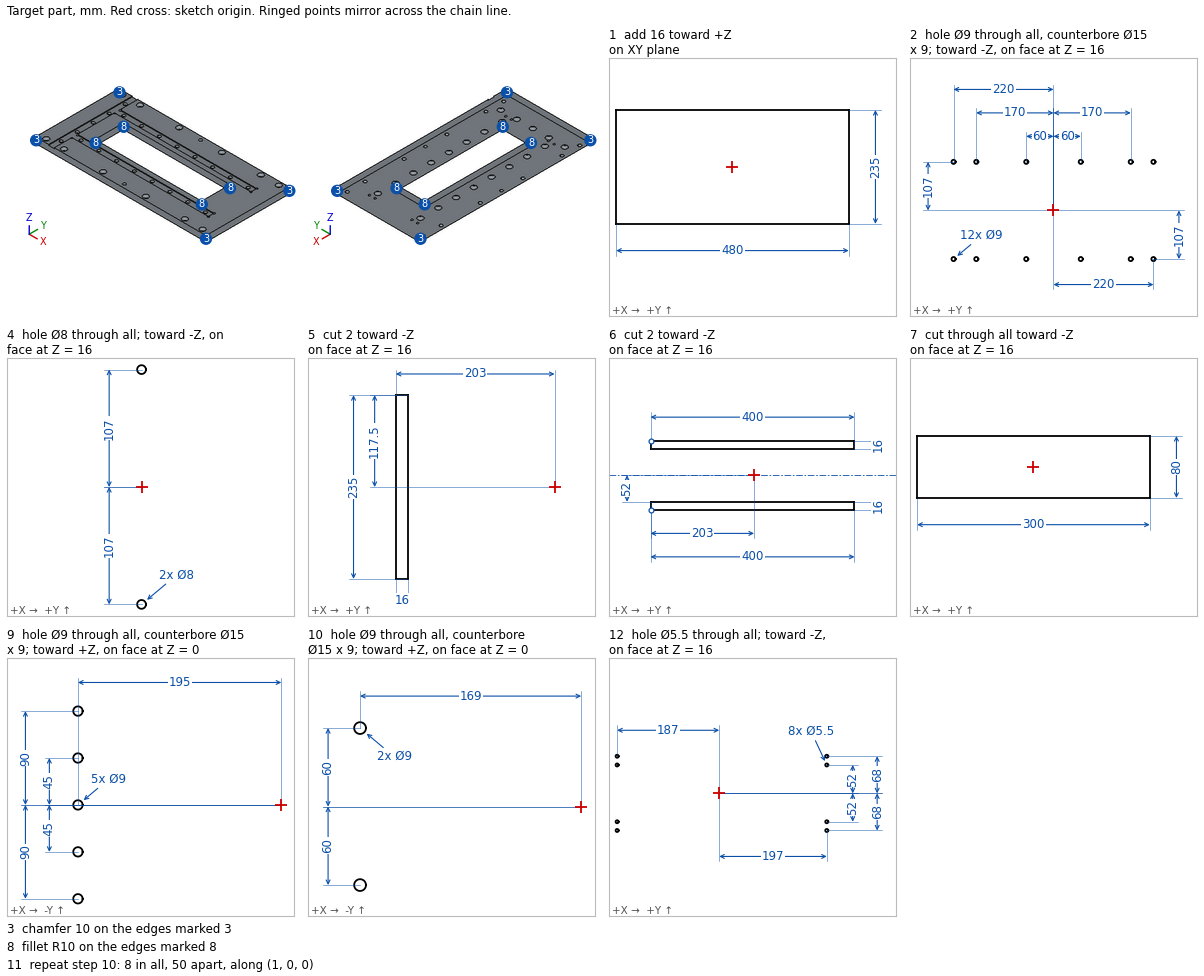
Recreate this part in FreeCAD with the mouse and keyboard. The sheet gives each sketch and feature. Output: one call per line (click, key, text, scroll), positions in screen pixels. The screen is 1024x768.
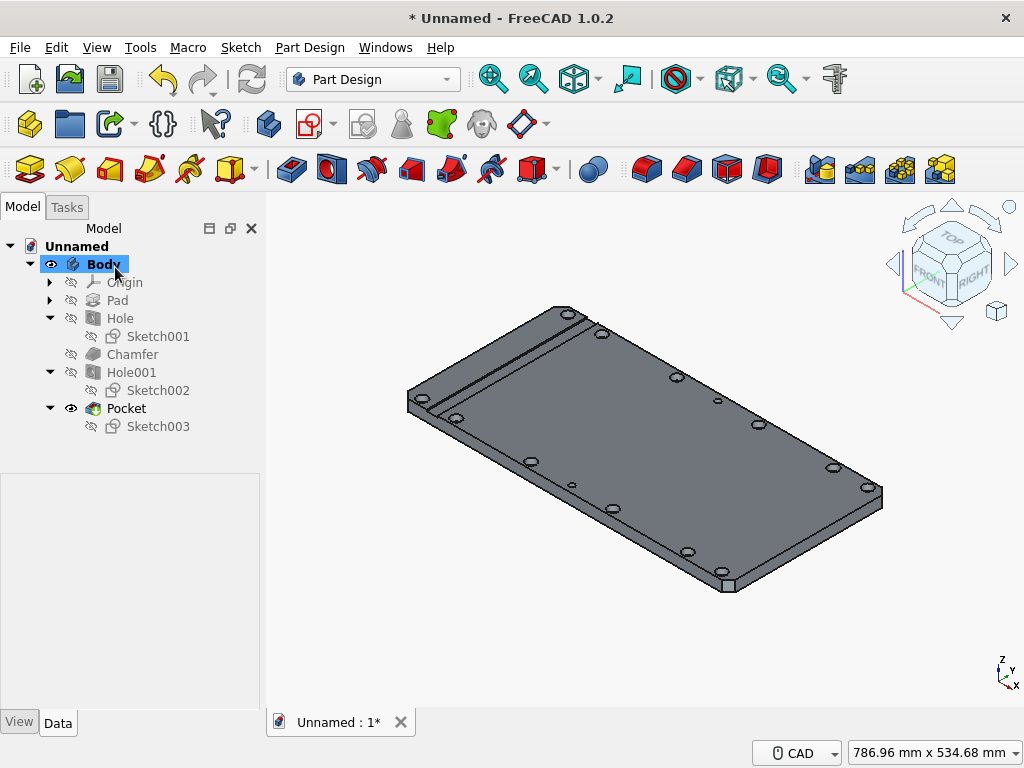
click(663, 453)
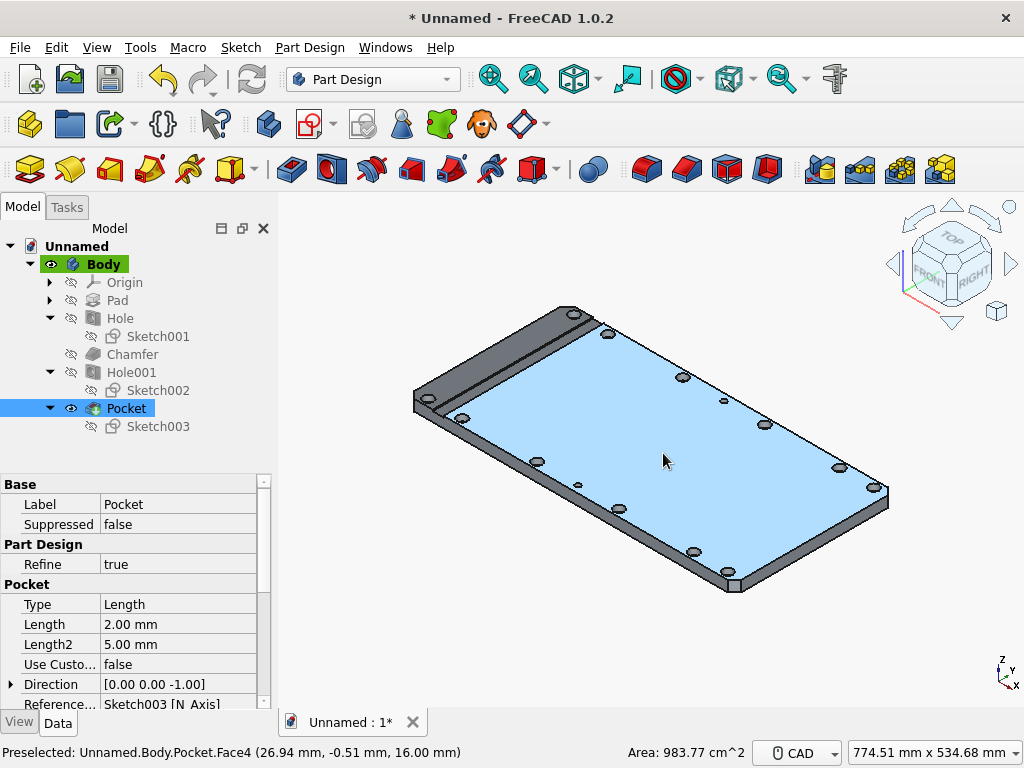
click(310, 124)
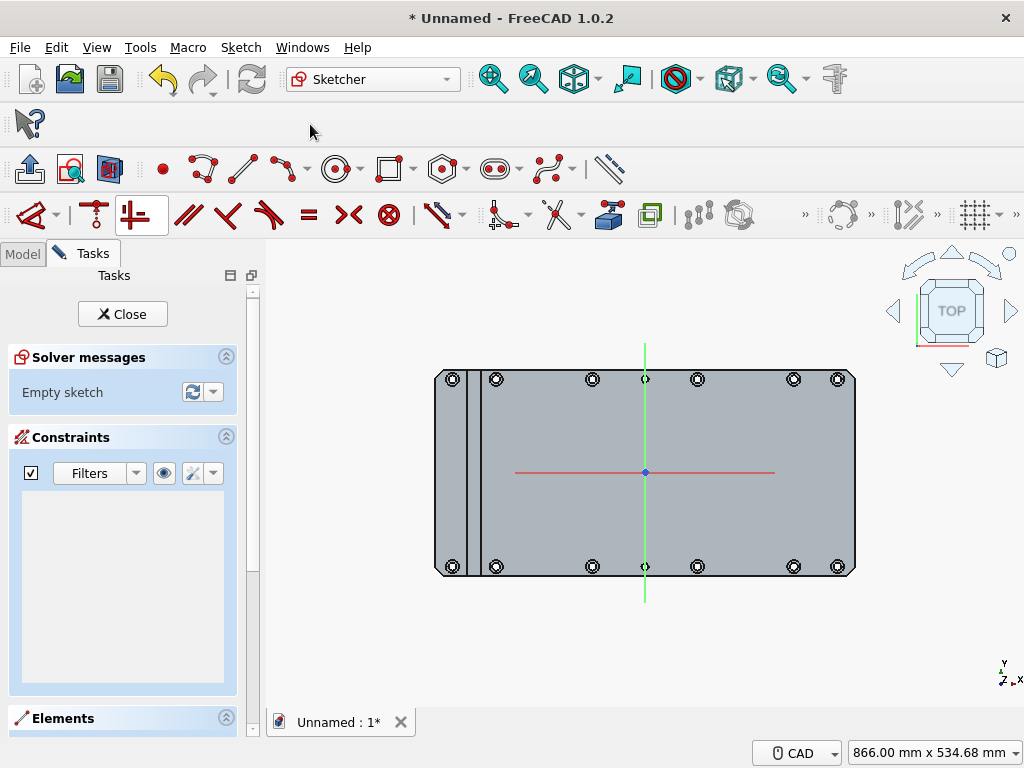
click(390, 170)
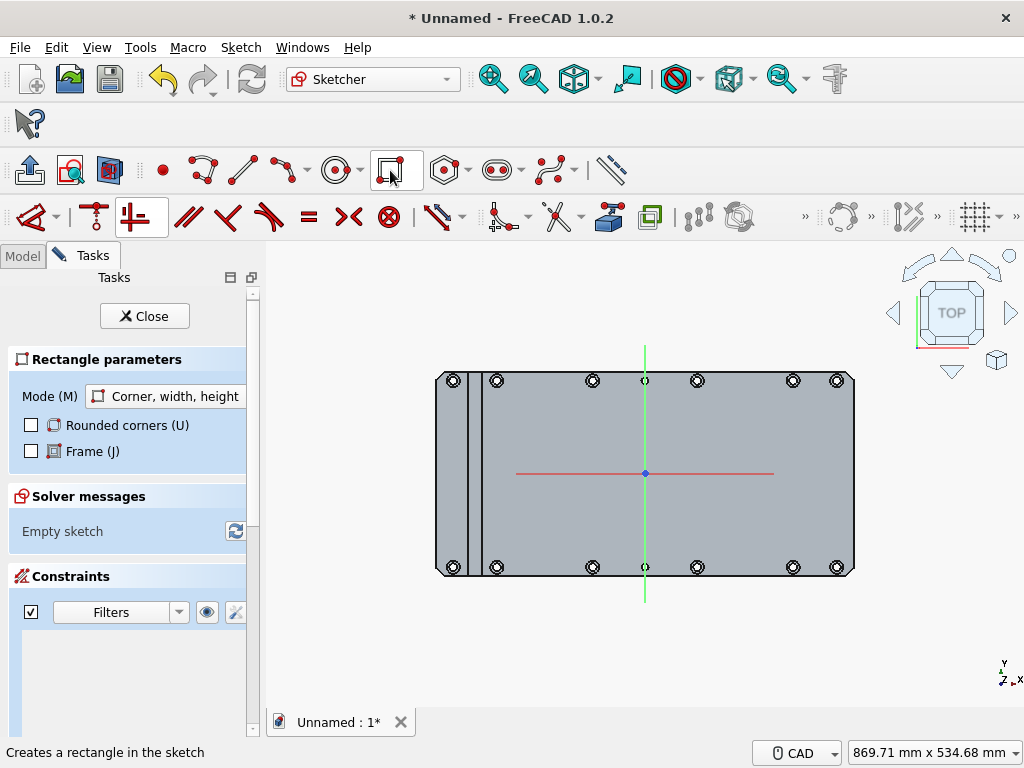
click(468, 519)
move(817, 533)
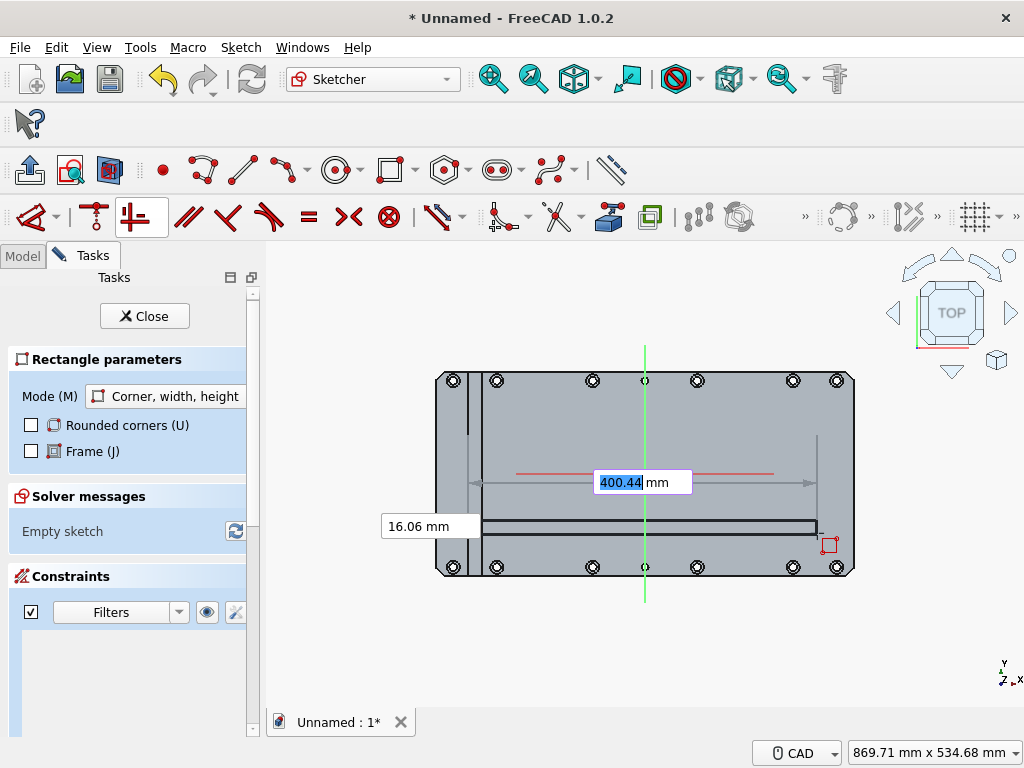
text(400)
key(Tab)
text(16)
key(Return)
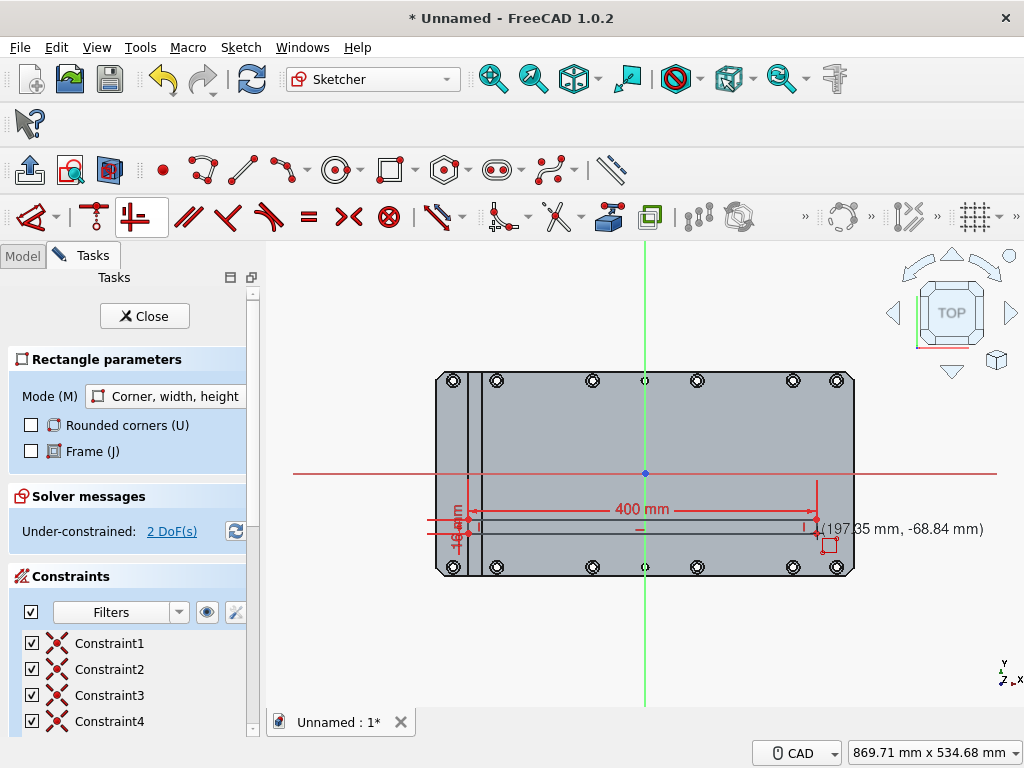
click(468, 415)
move(817, 429)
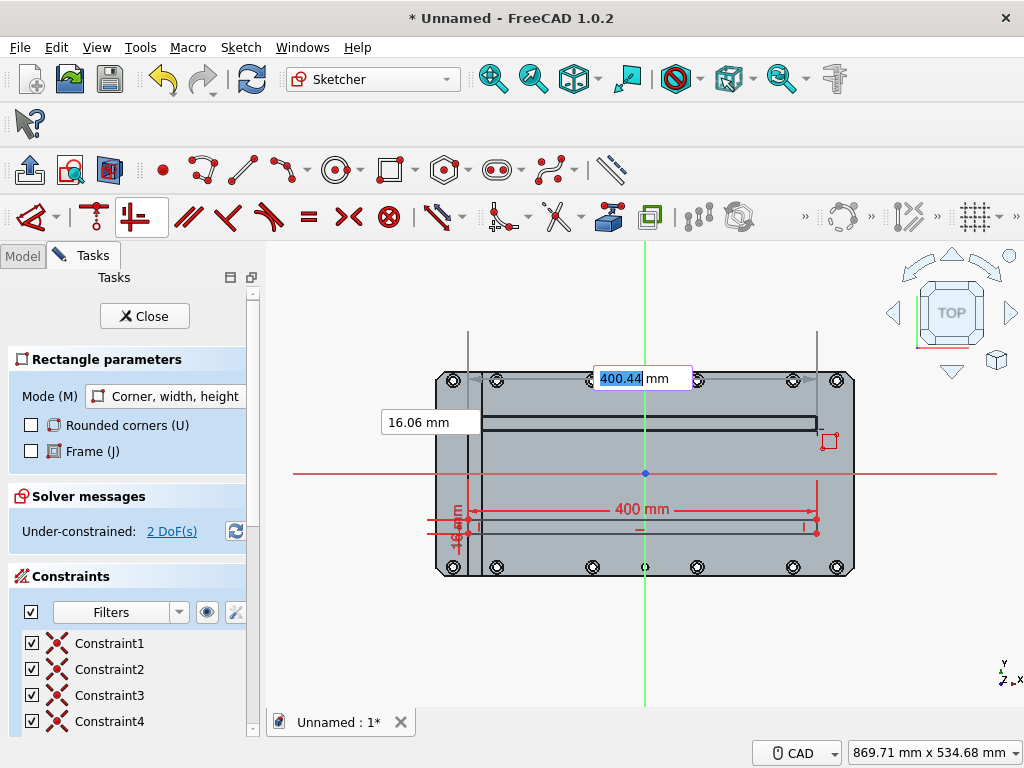
text(400)
key(Tab)
text(16)
key(Return)
key(Escape)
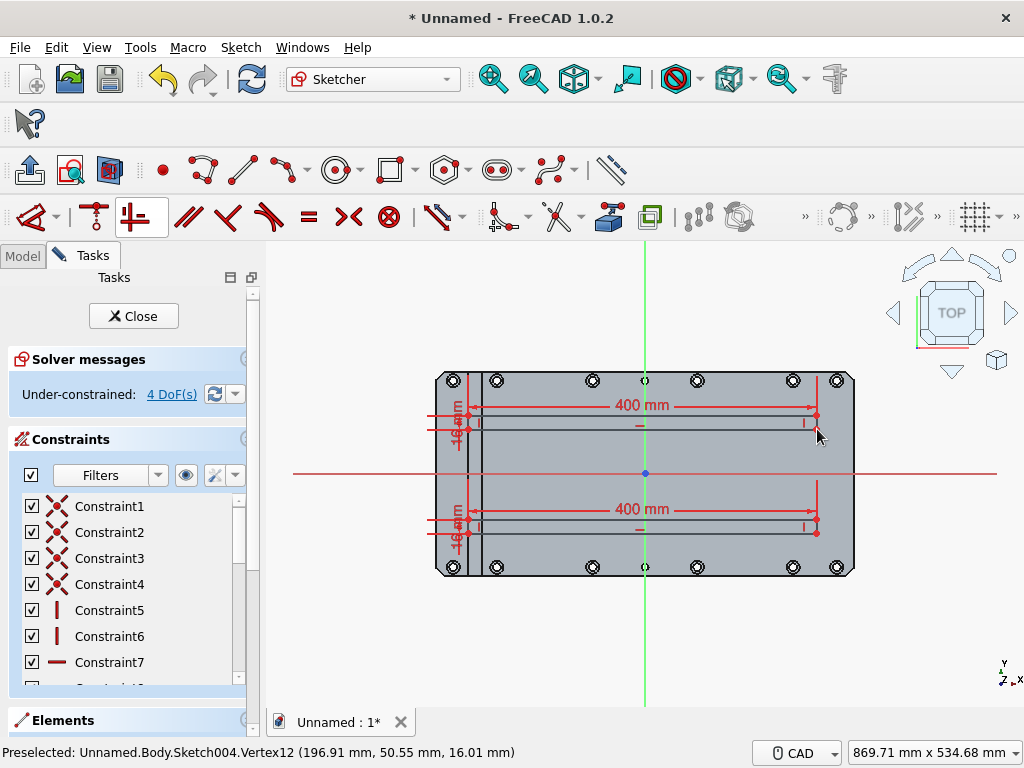
click(468, 534)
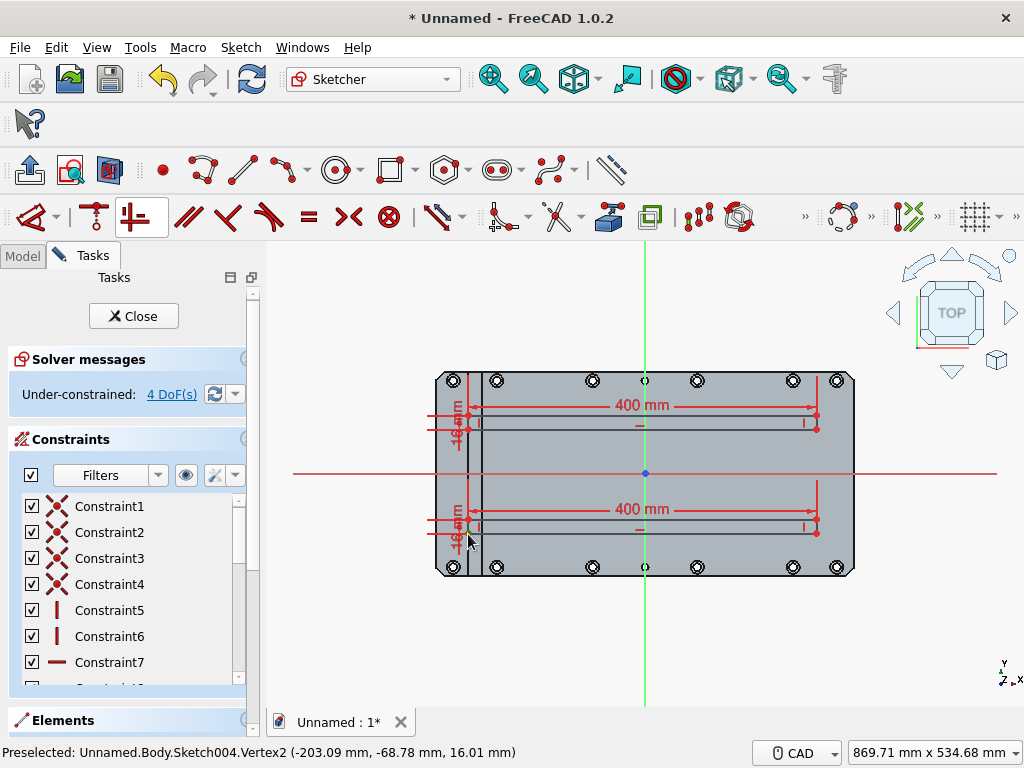
click(468, 416)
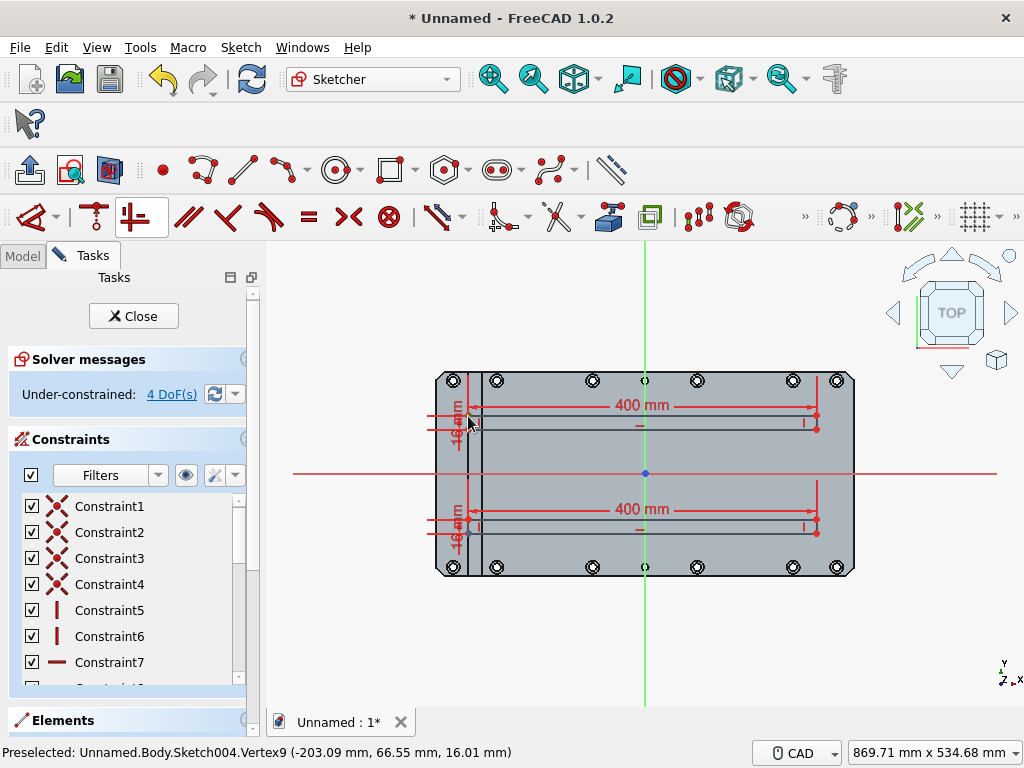
click(334, 474)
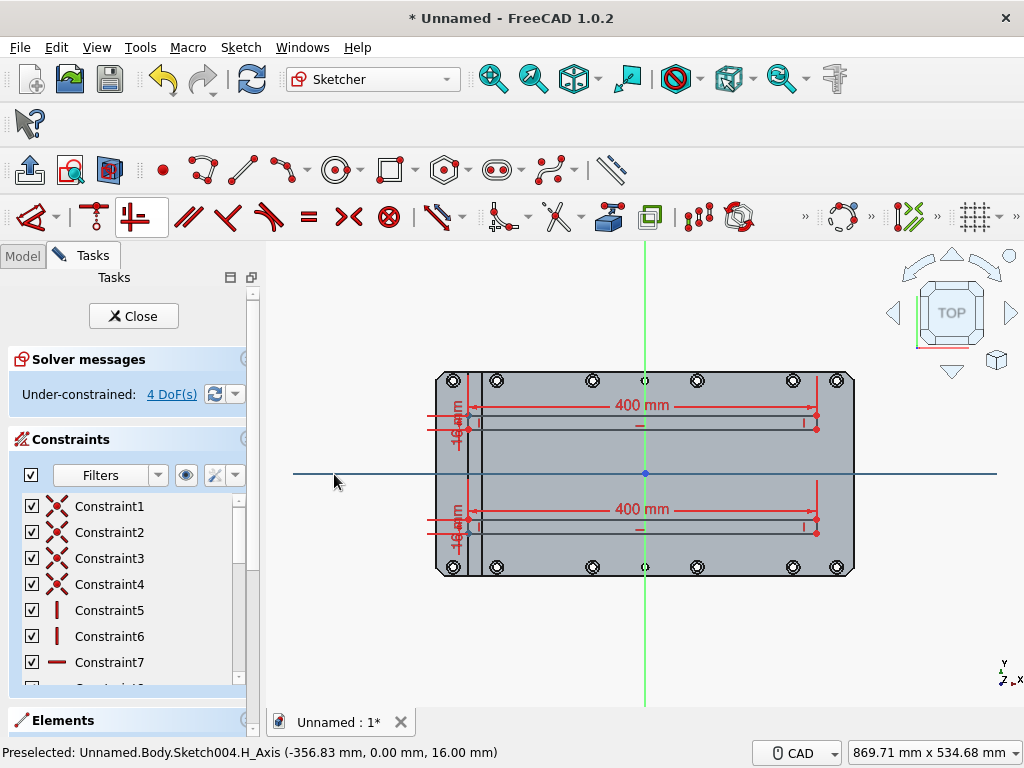
click(350, 218)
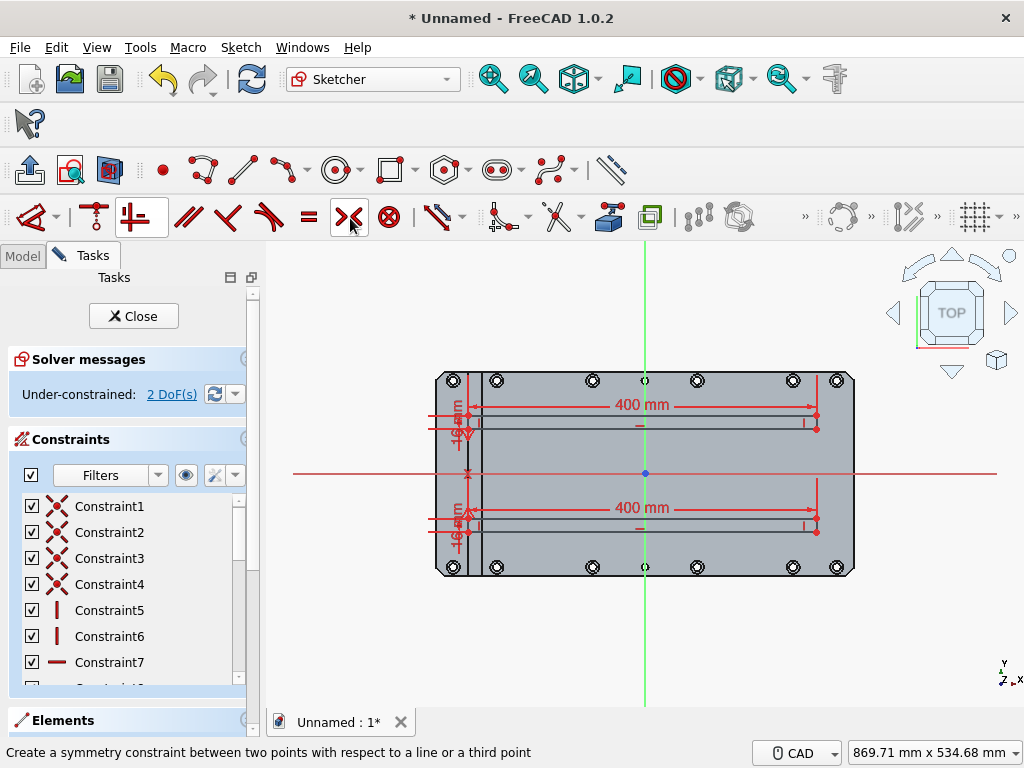
click(32, 218)